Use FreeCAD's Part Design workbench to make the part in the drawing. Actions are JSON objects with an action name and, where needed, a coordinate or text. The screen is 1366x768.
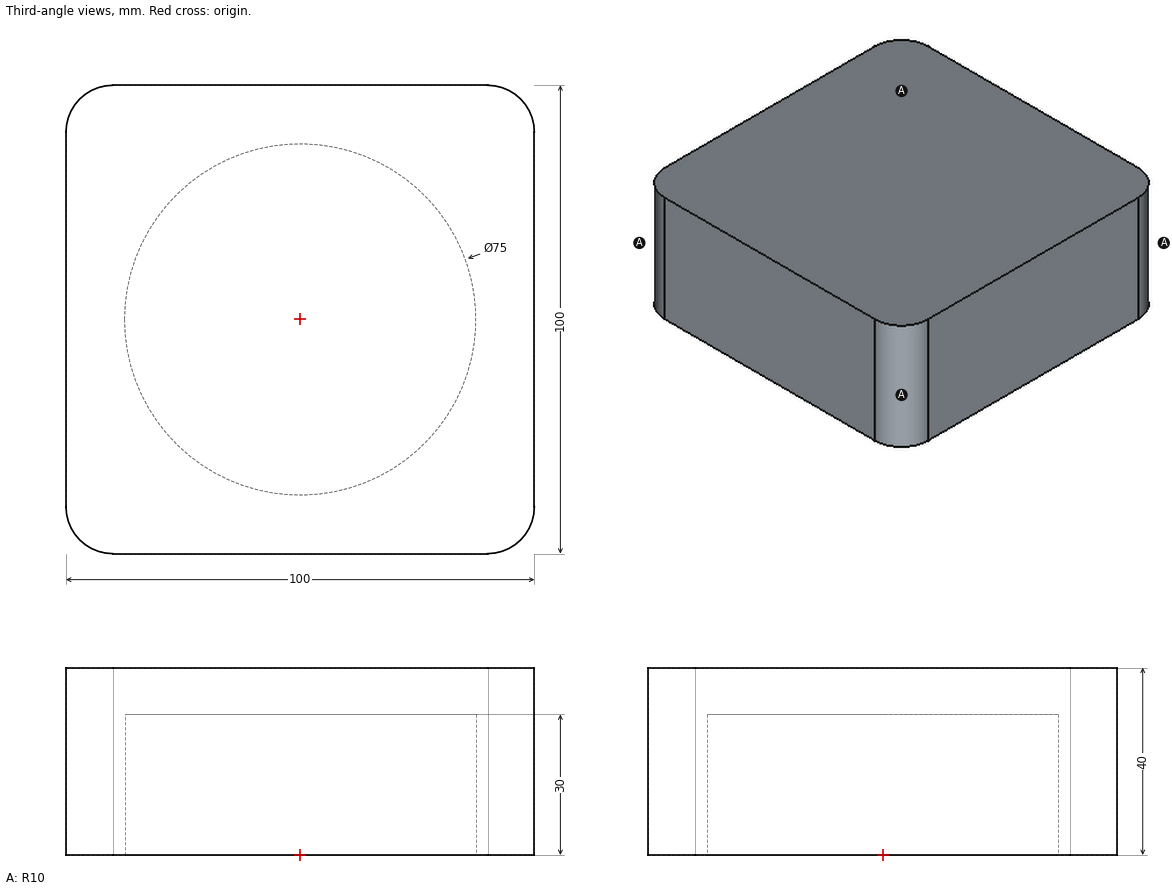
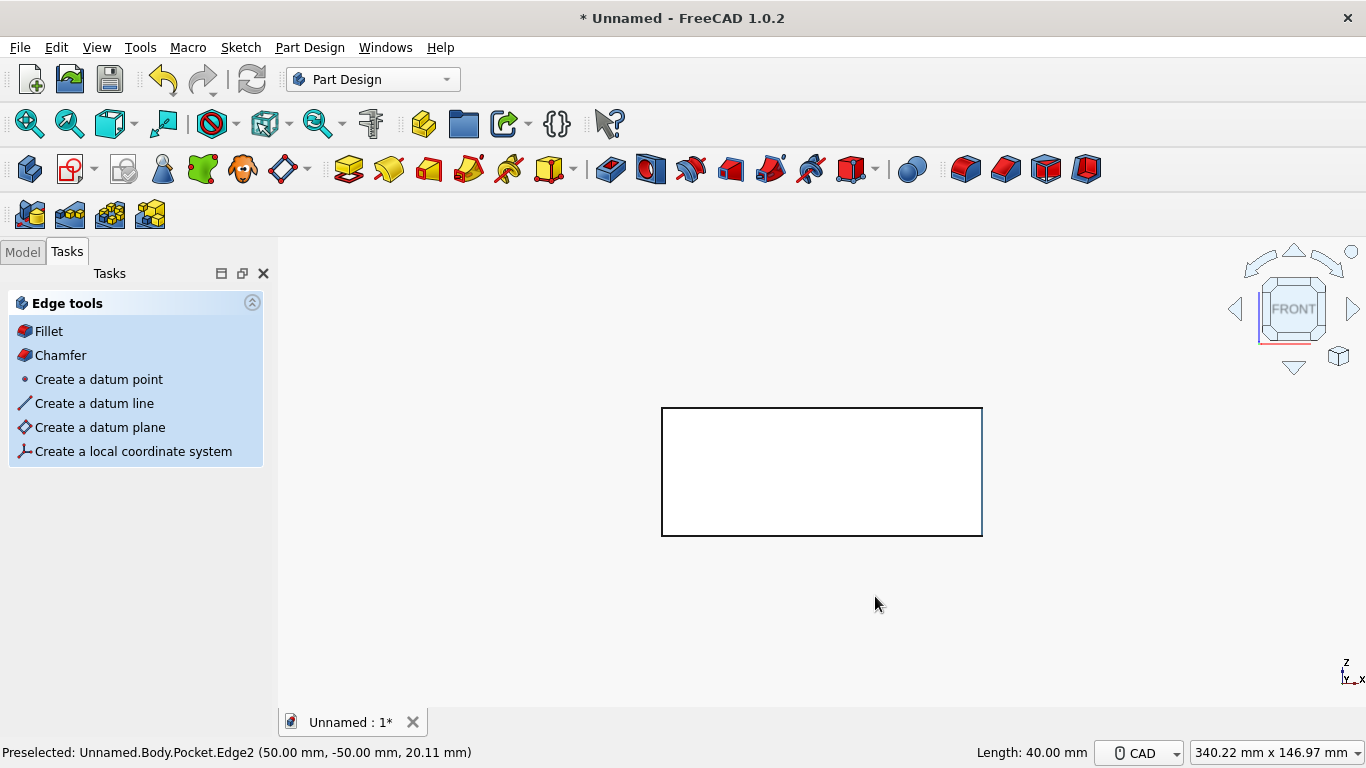
{"action": "key", "text": "v f"}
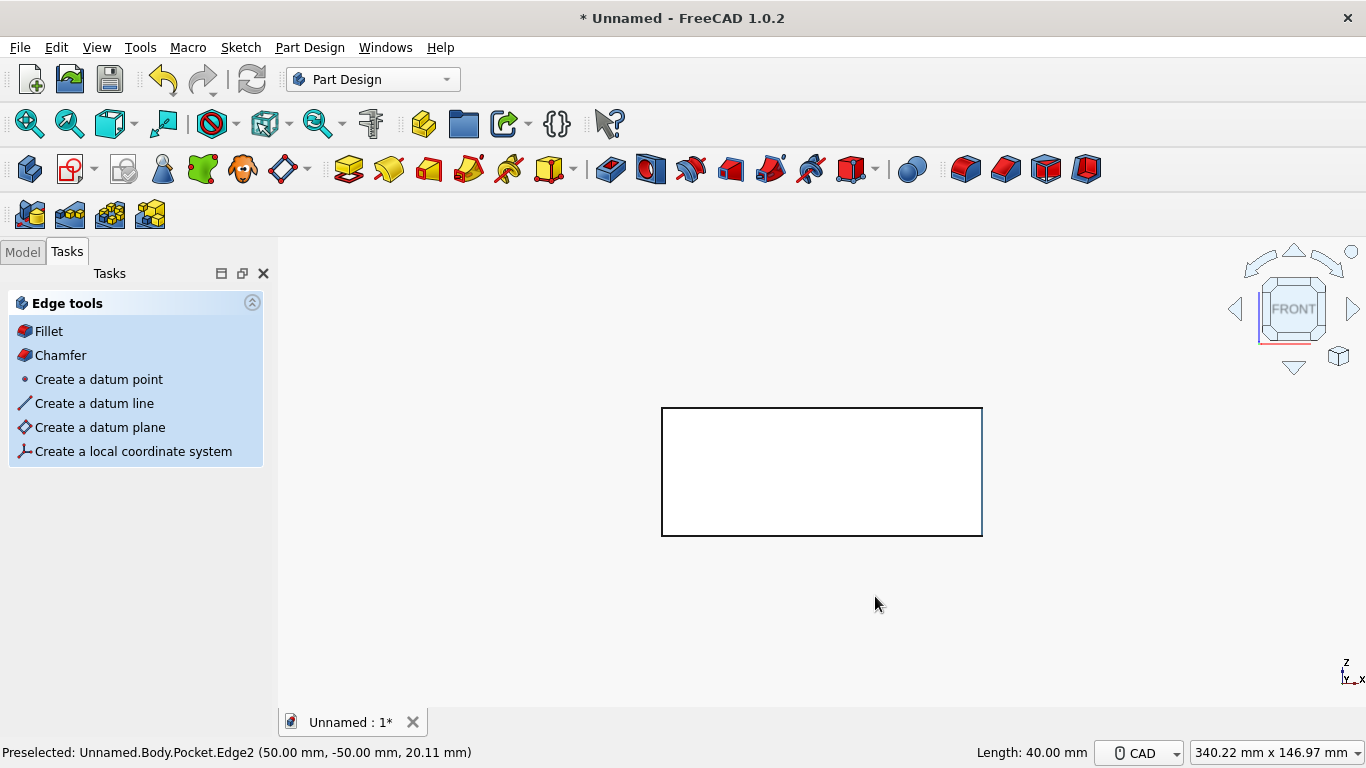
{"action": "left_click", "coordinate": [662, 471], "text": "ctrl"}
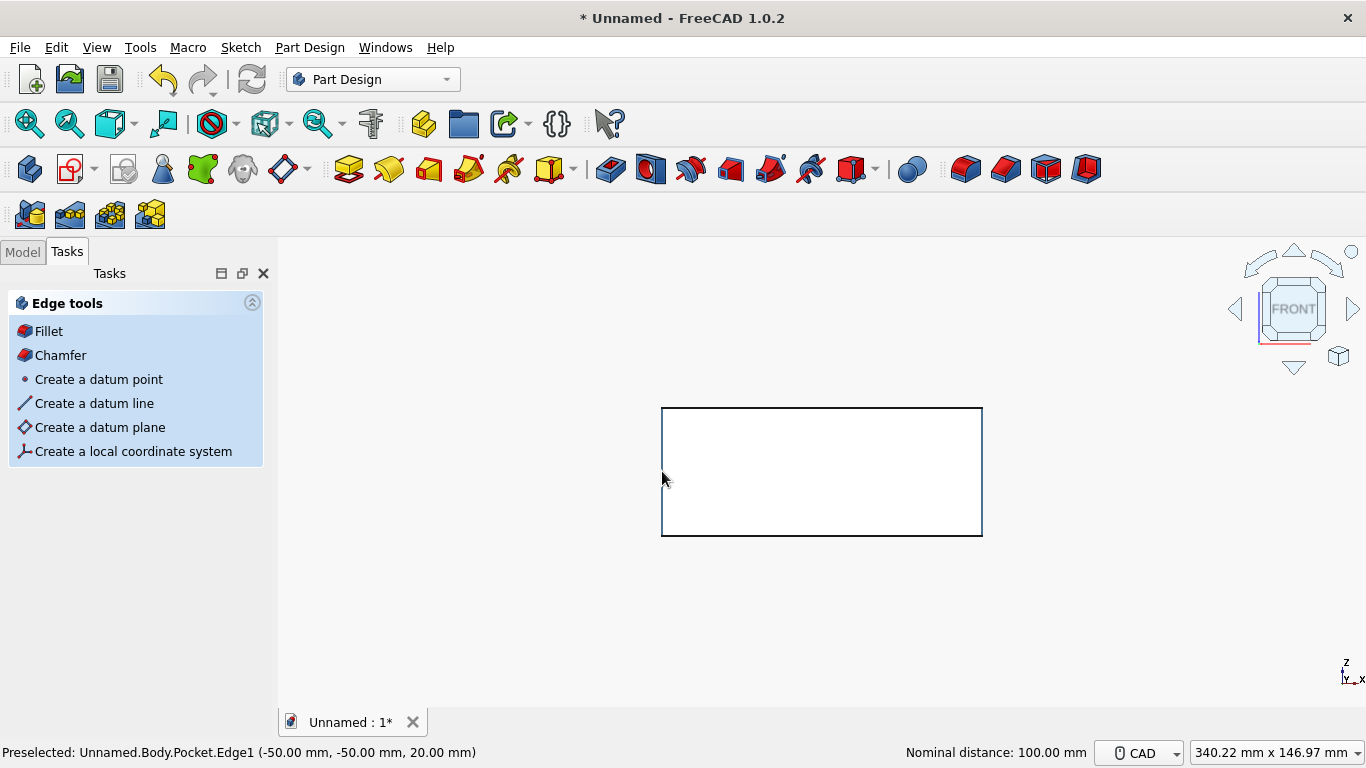
{"action": "key", "text": "3"}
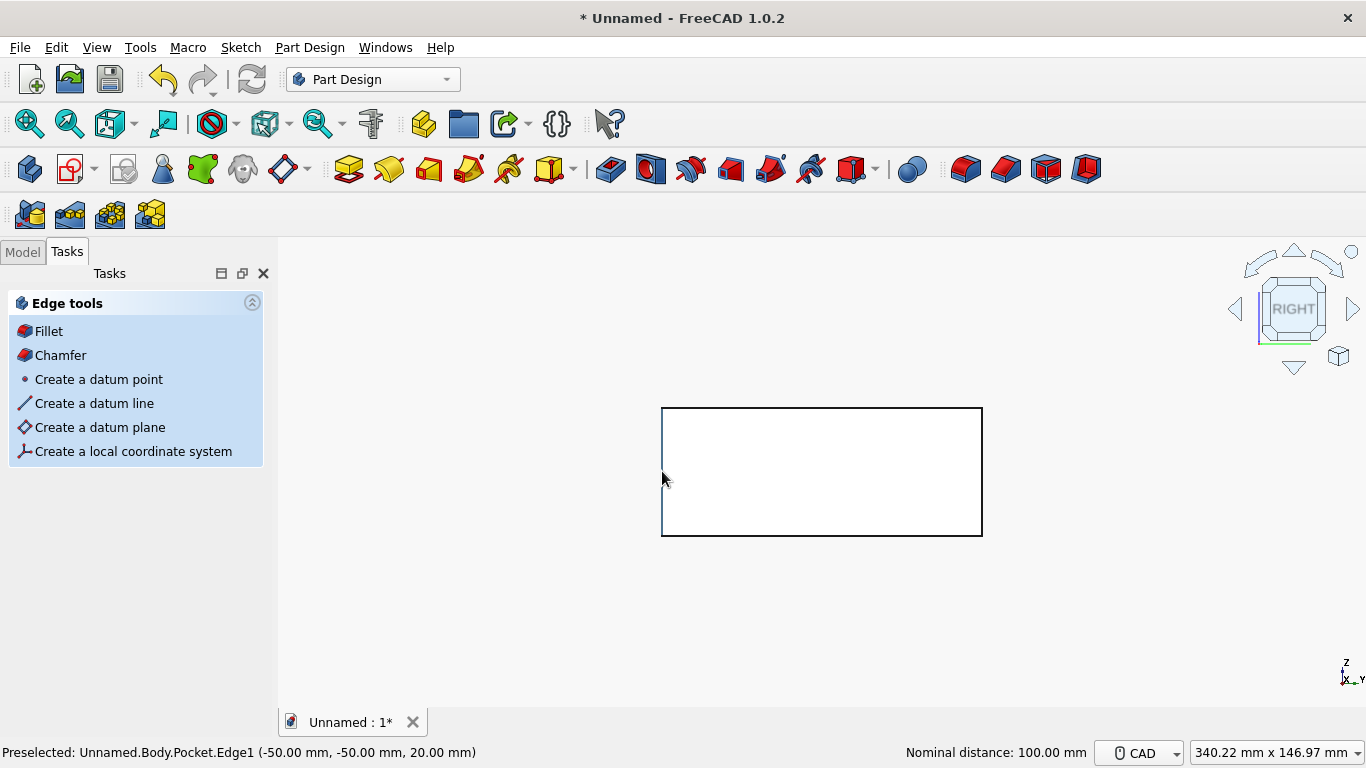
{"action": "left_click", "coordinate": [30, 124]}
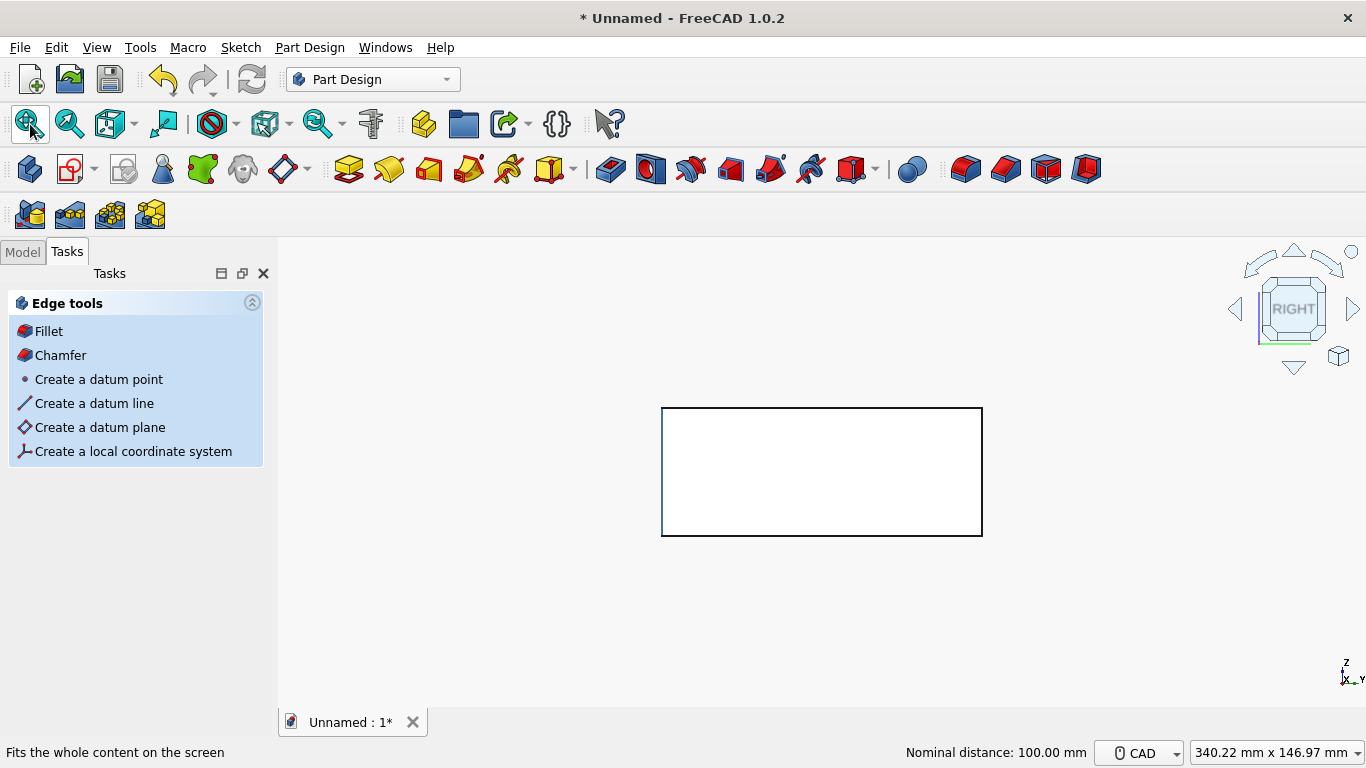
{"action": "left_click", "coordinate": [982, 471], "text": "ctrl"}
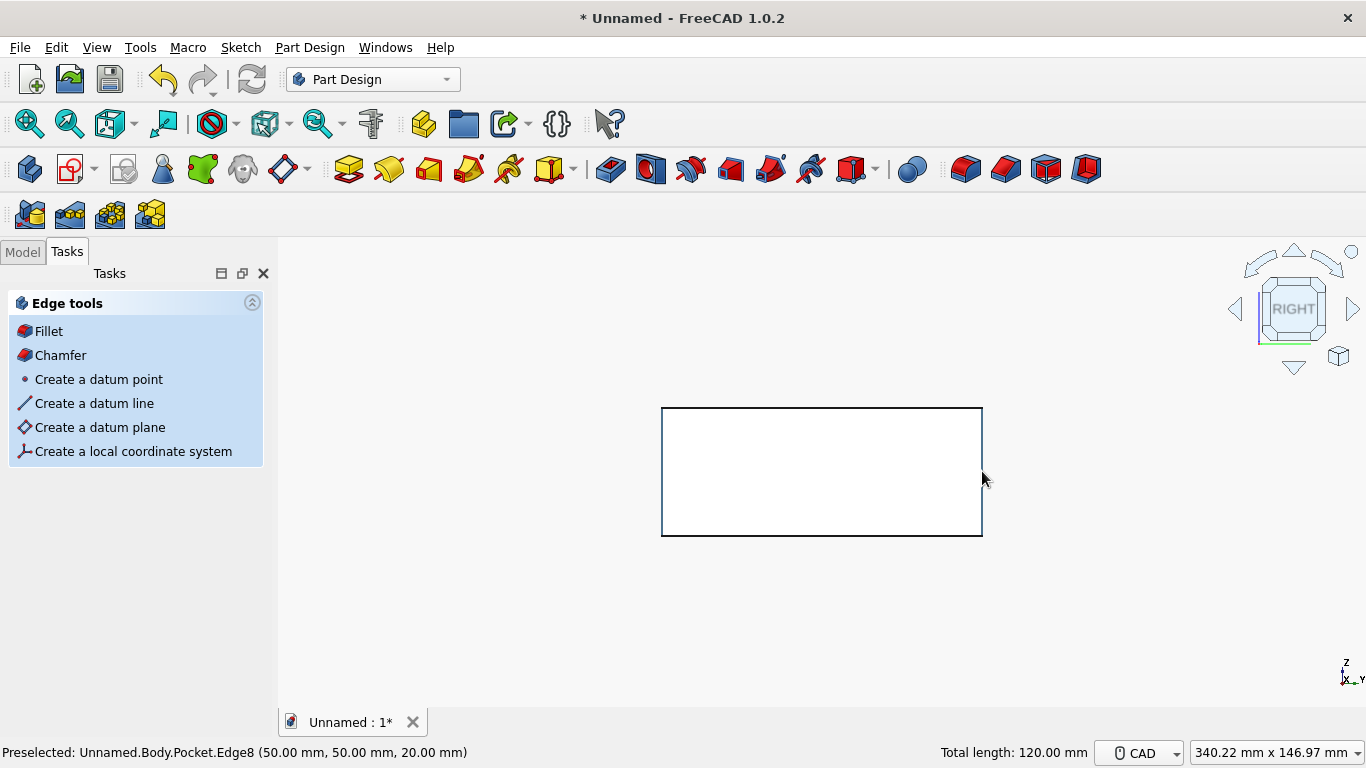
{"action": "key", "text": "5"}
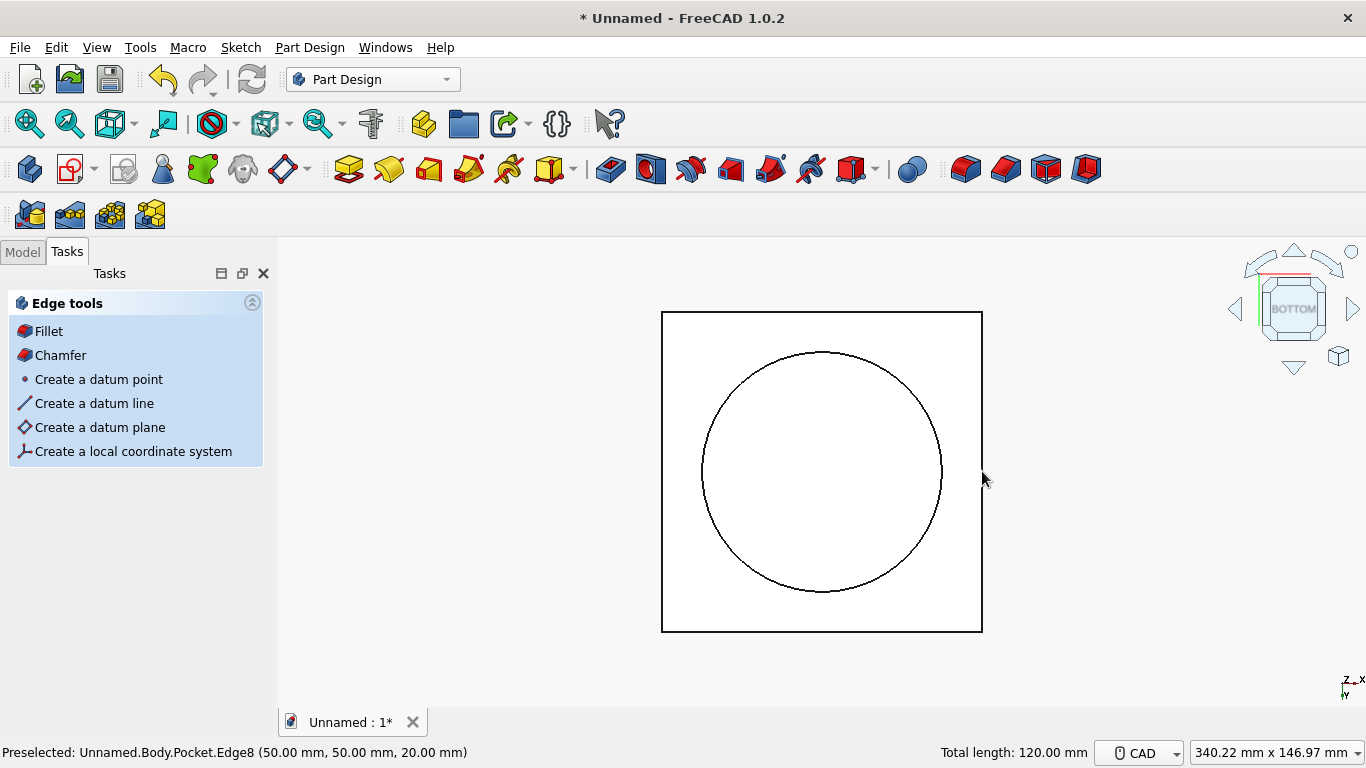
{"action": "key", "text": "4"}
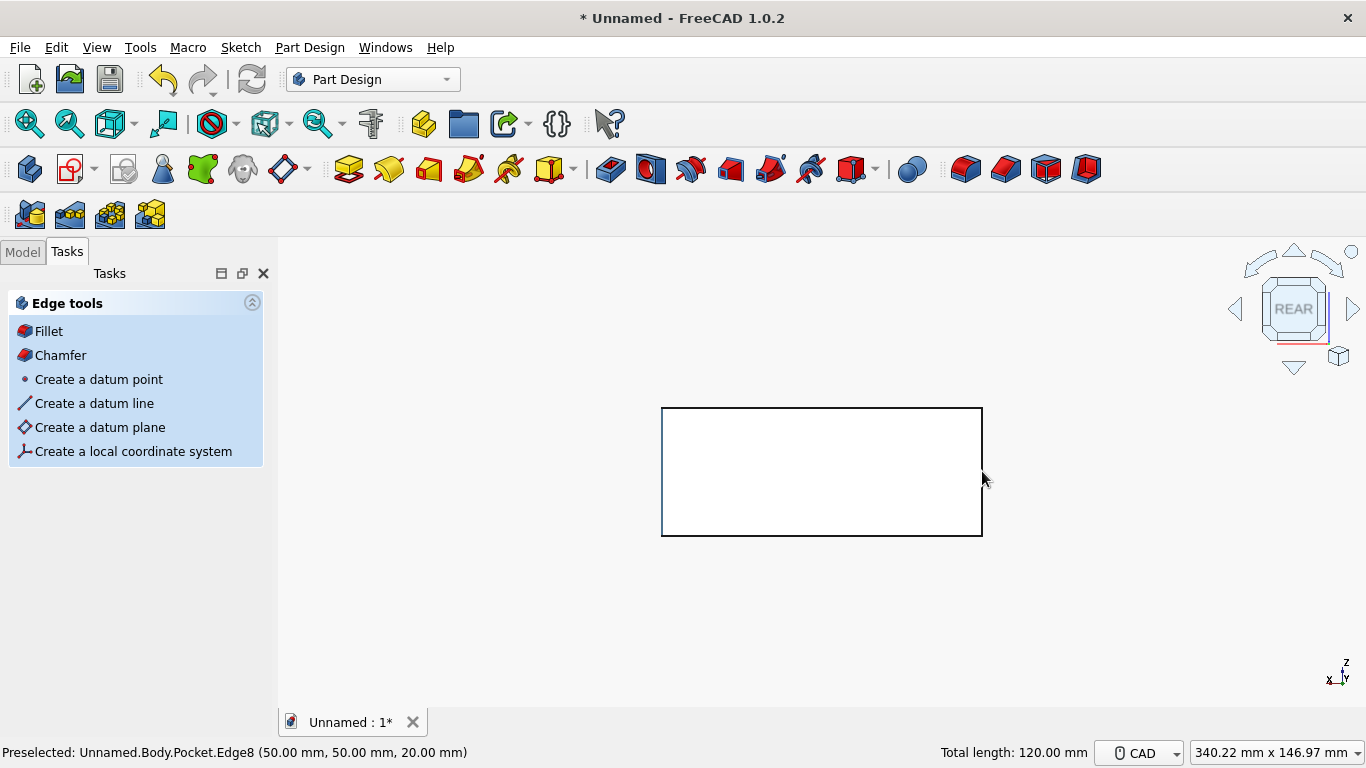
{"action": "left_click", "coordinate": [30, 124]}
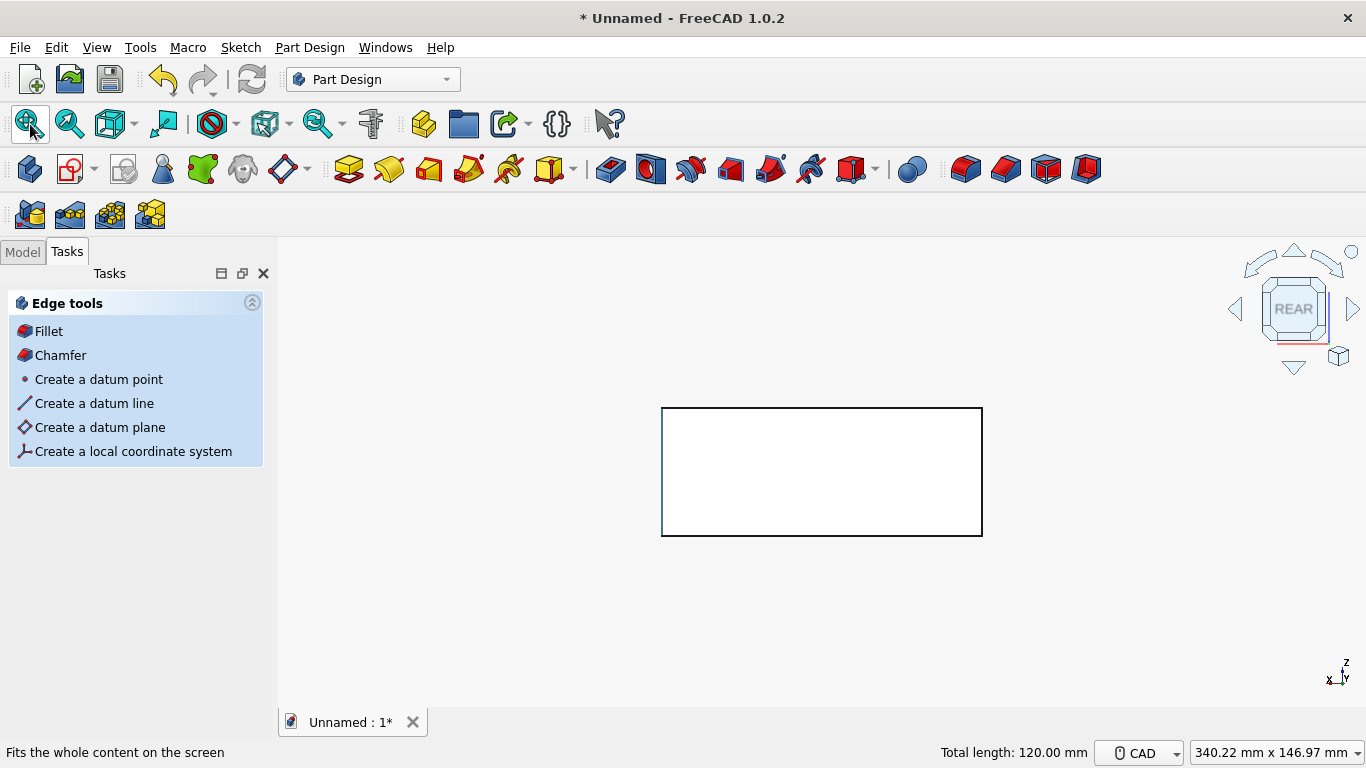
{"action": "left_click", "coordinate": [982, 471], "text": "ctrl"}